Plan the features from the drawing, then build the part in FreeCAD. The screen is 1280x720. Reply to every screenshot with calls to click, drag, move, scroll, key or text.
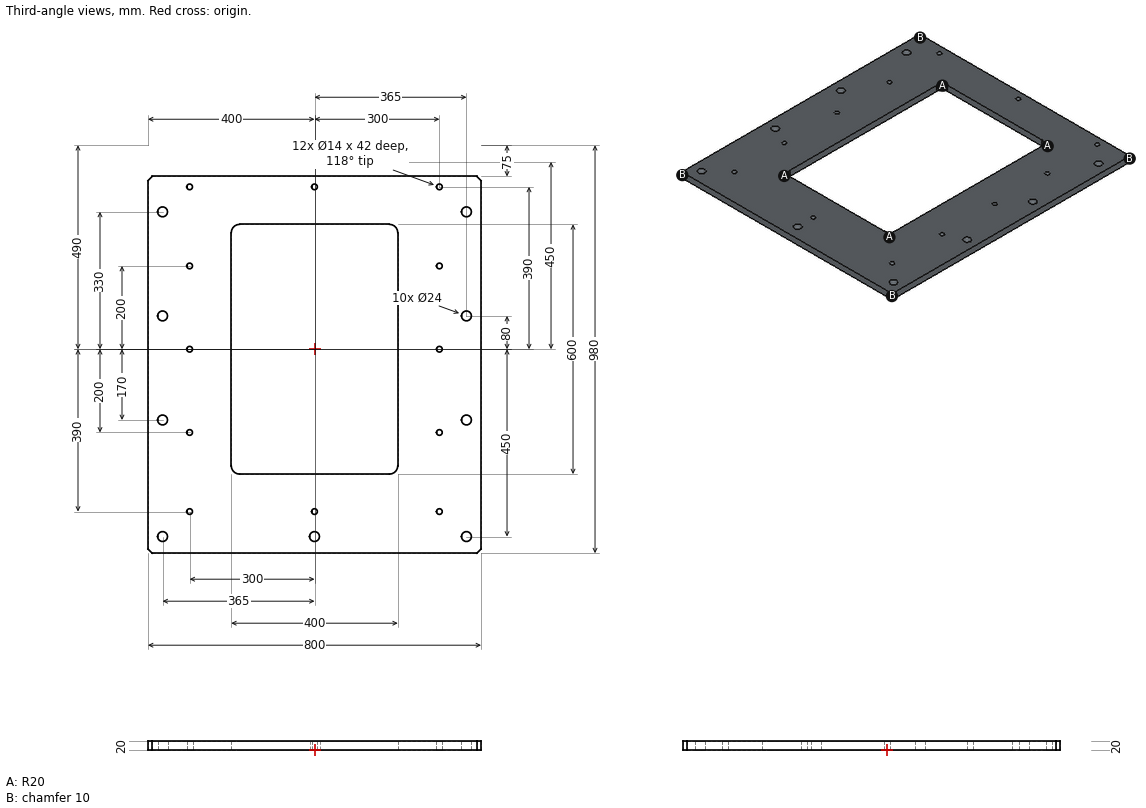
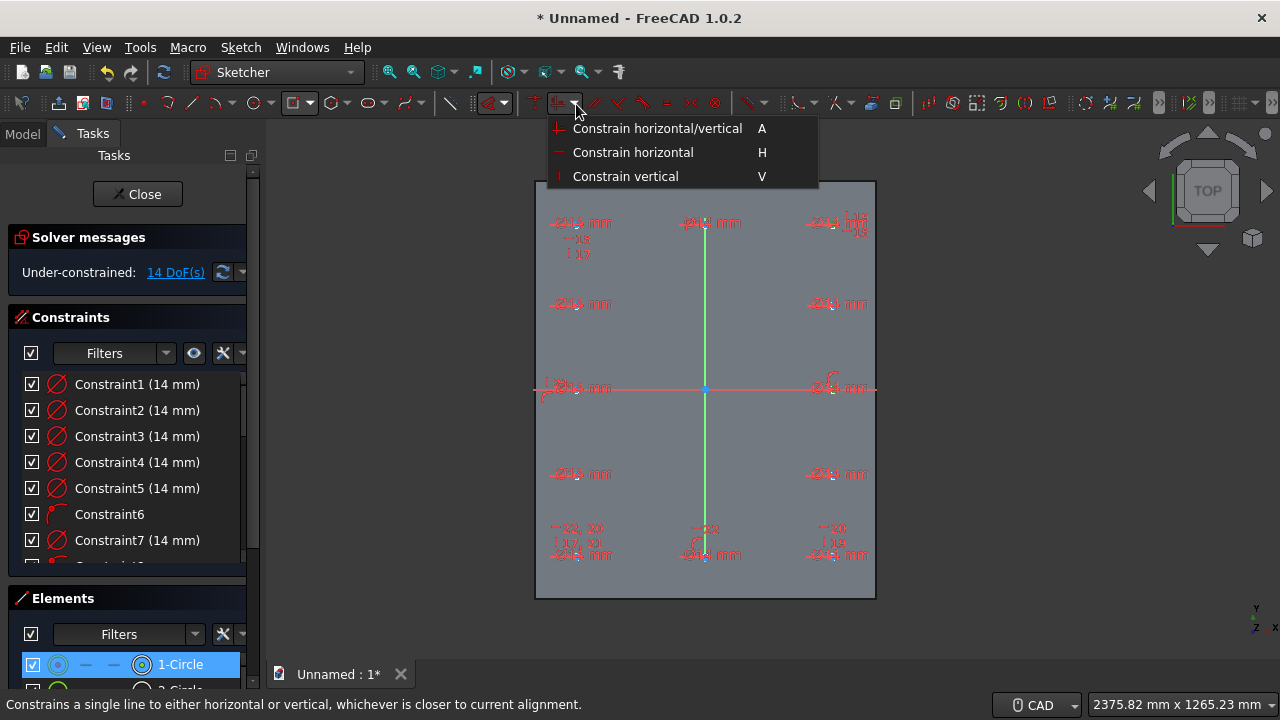
click(683, 176)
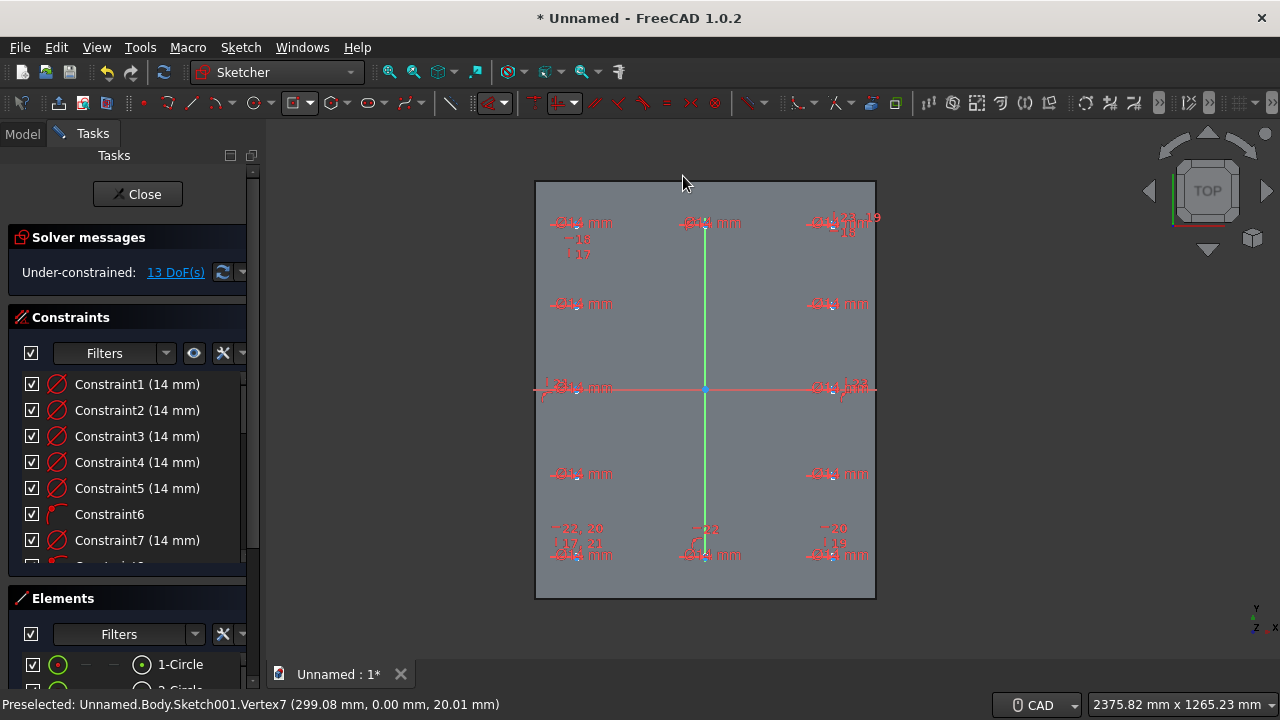
click(833, 225)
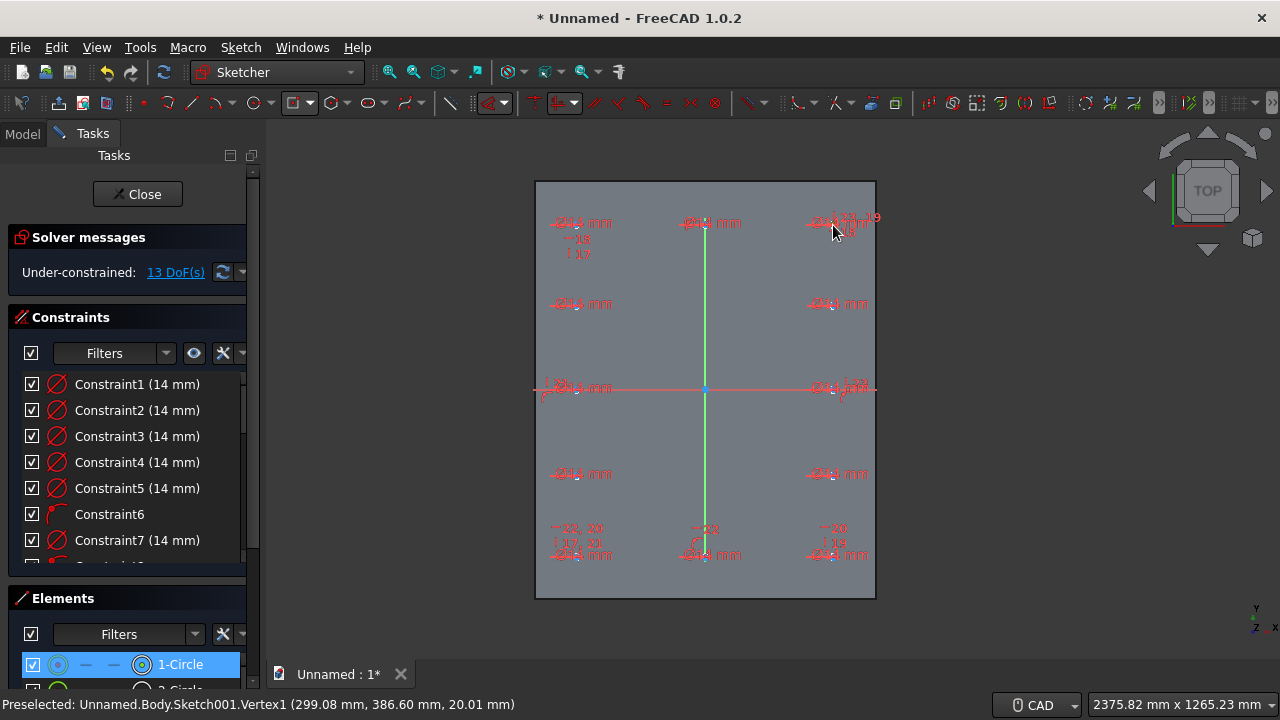
click(705, 225)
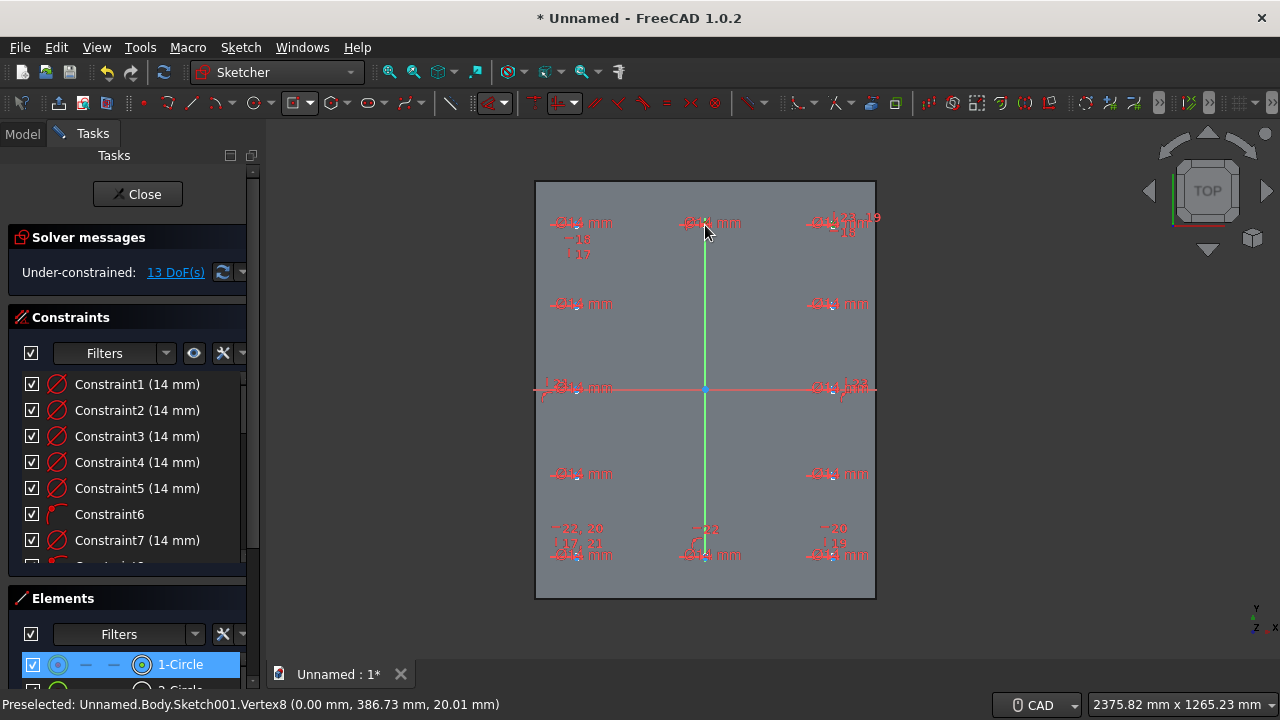
click(576, 104)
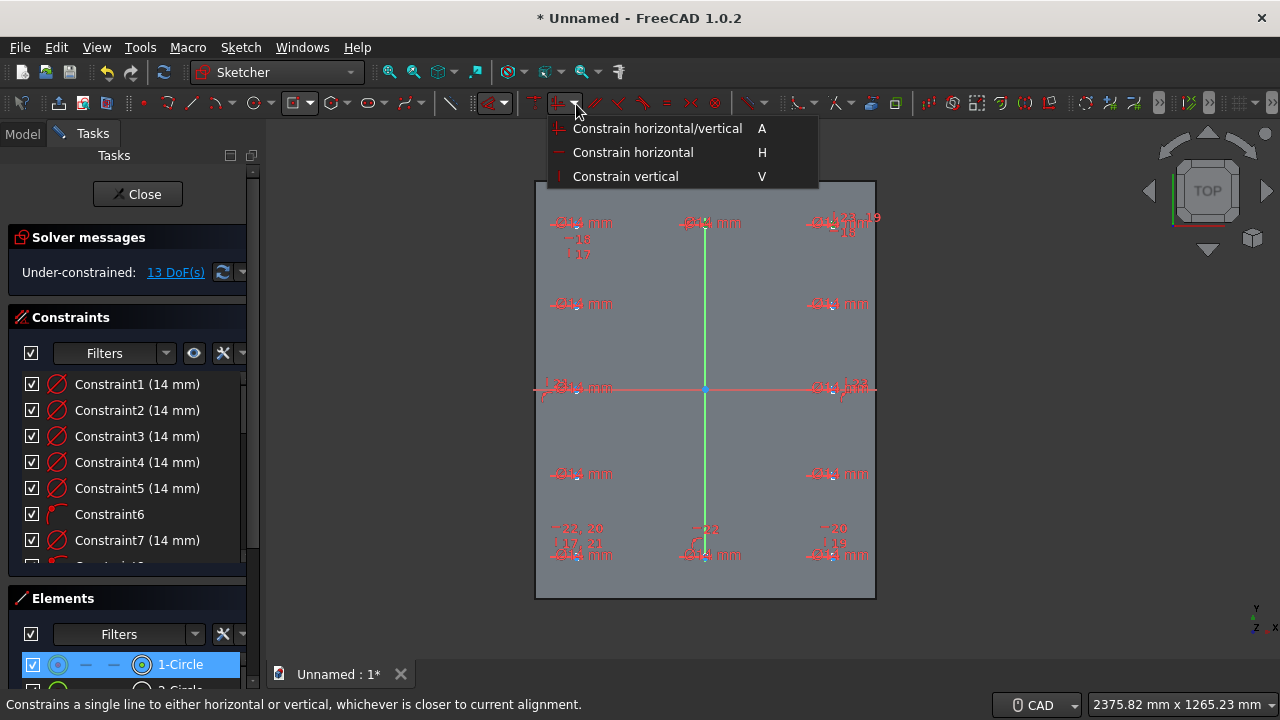
click(683, 152)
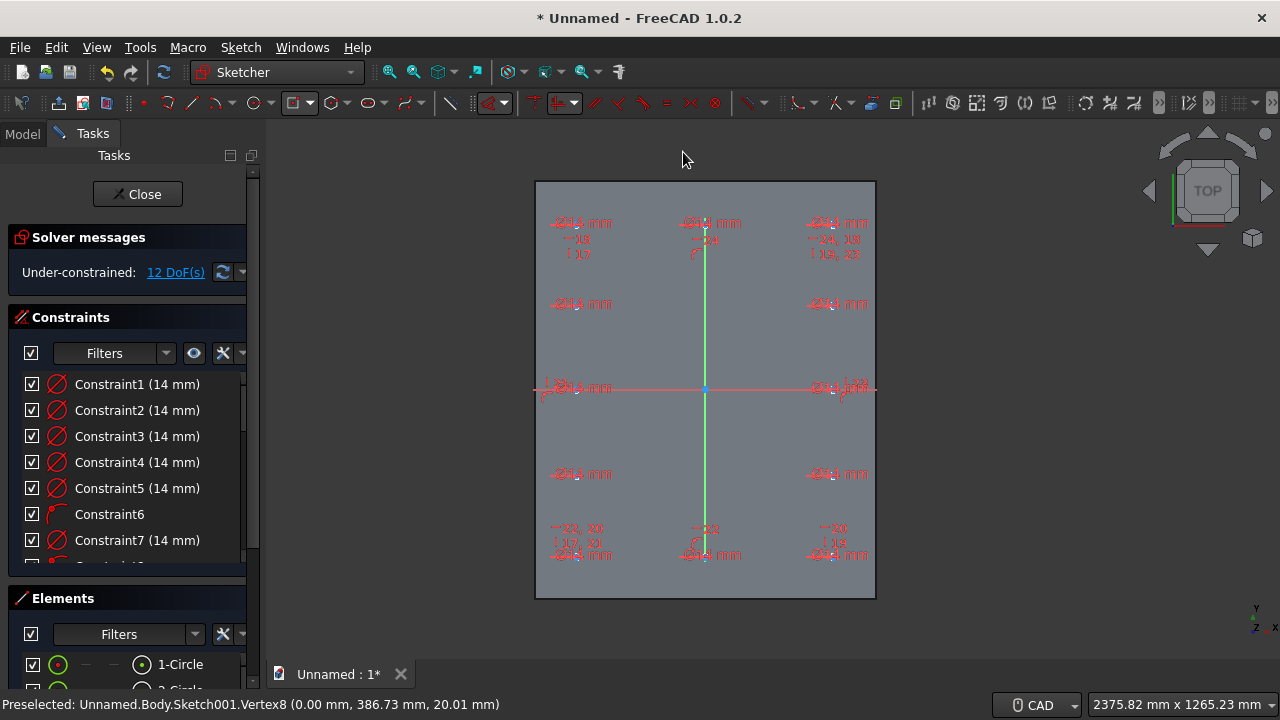
click(577, 225)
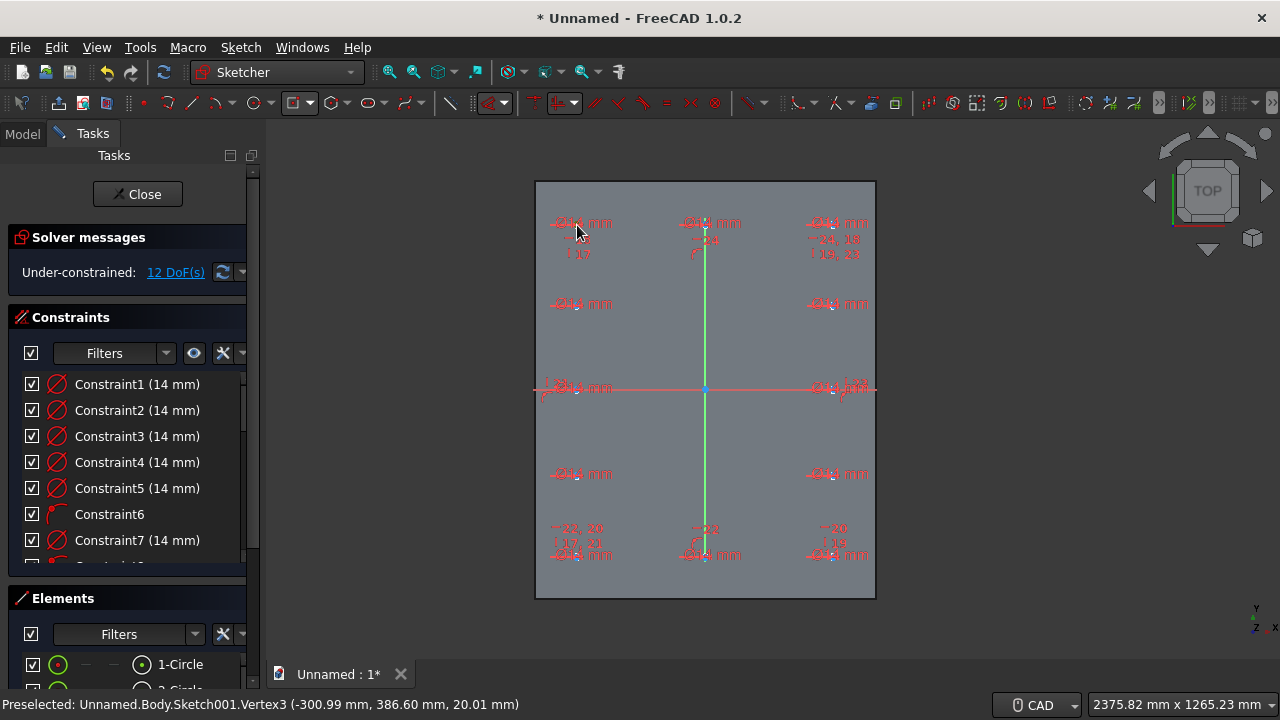
click(577, 306)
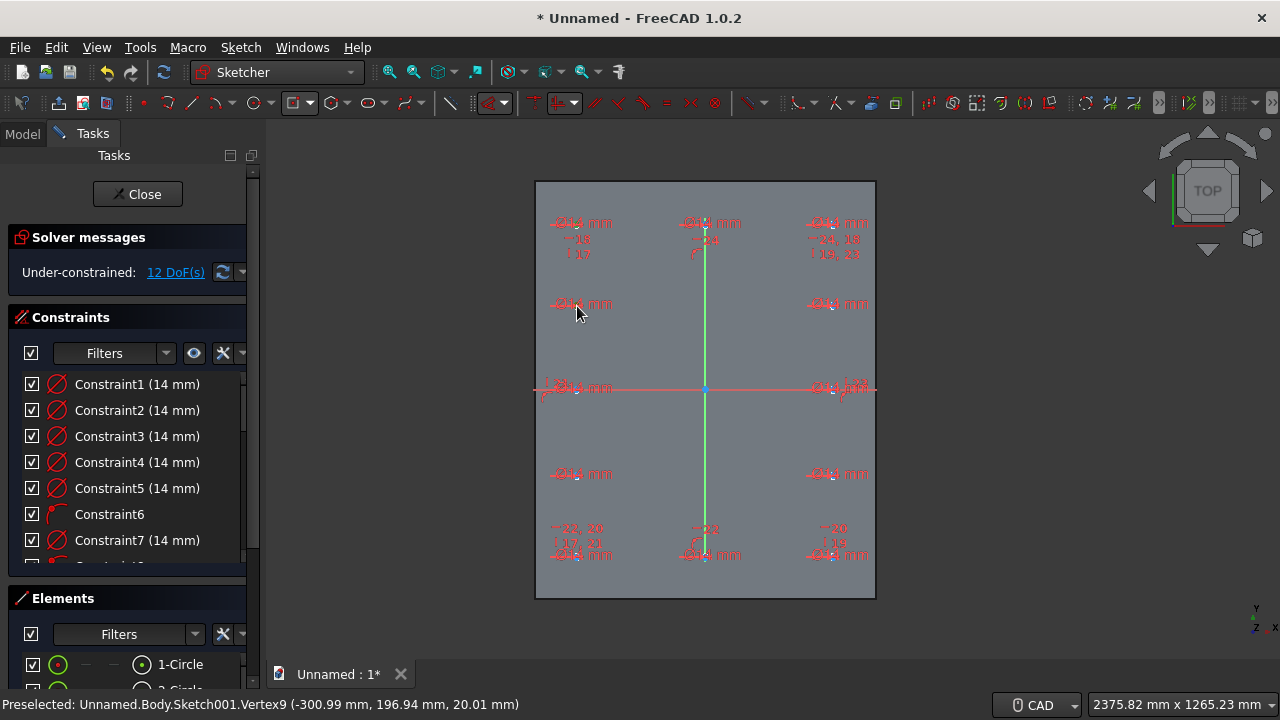
click(576, 104)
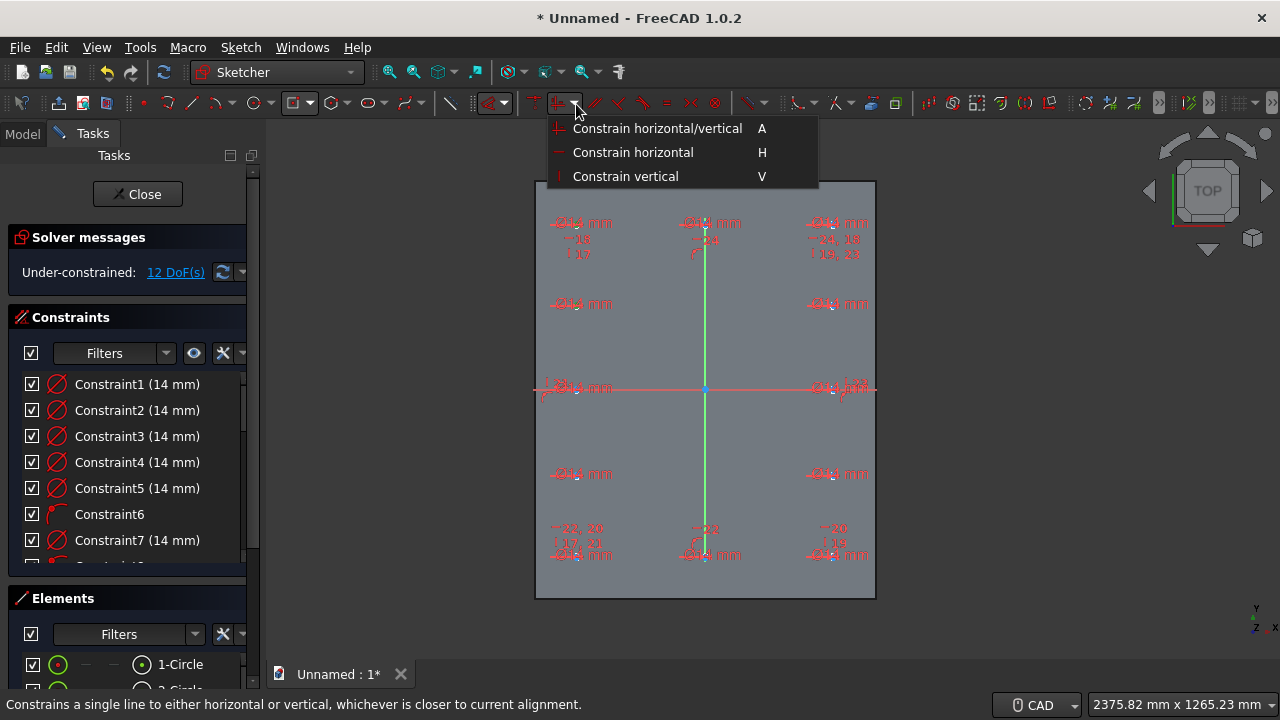
click(683, 176)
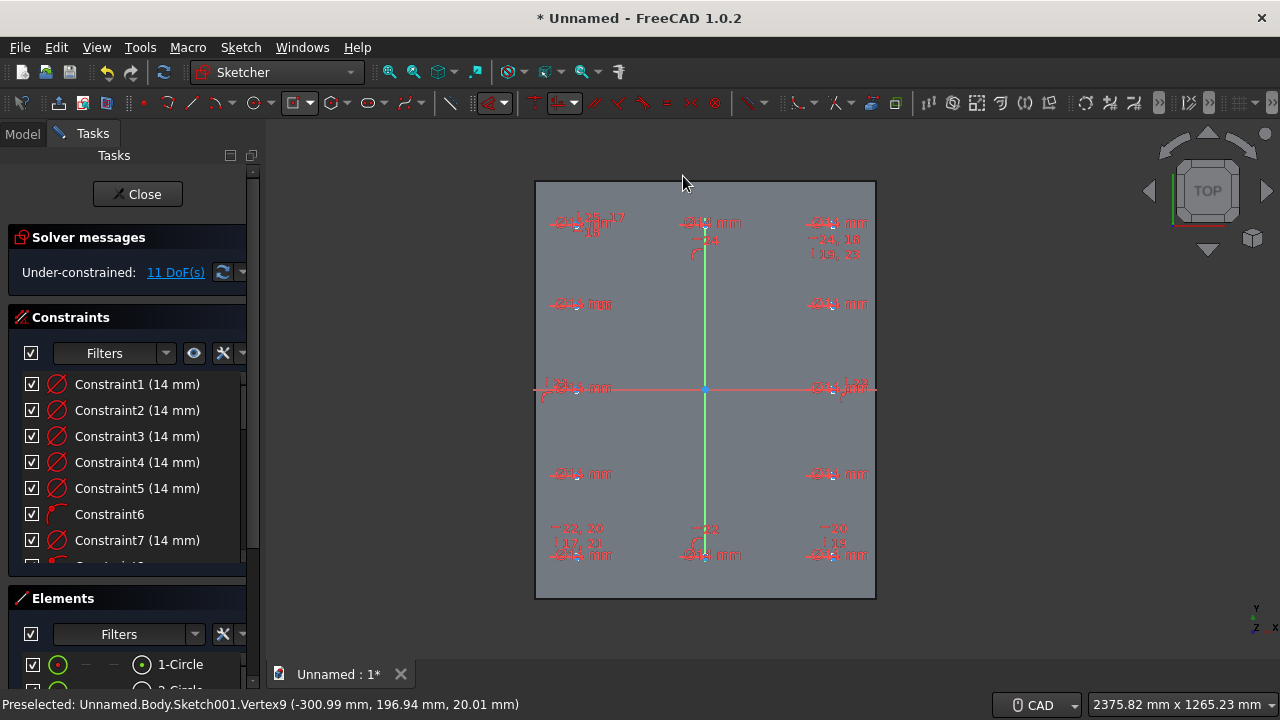
click(833, 225)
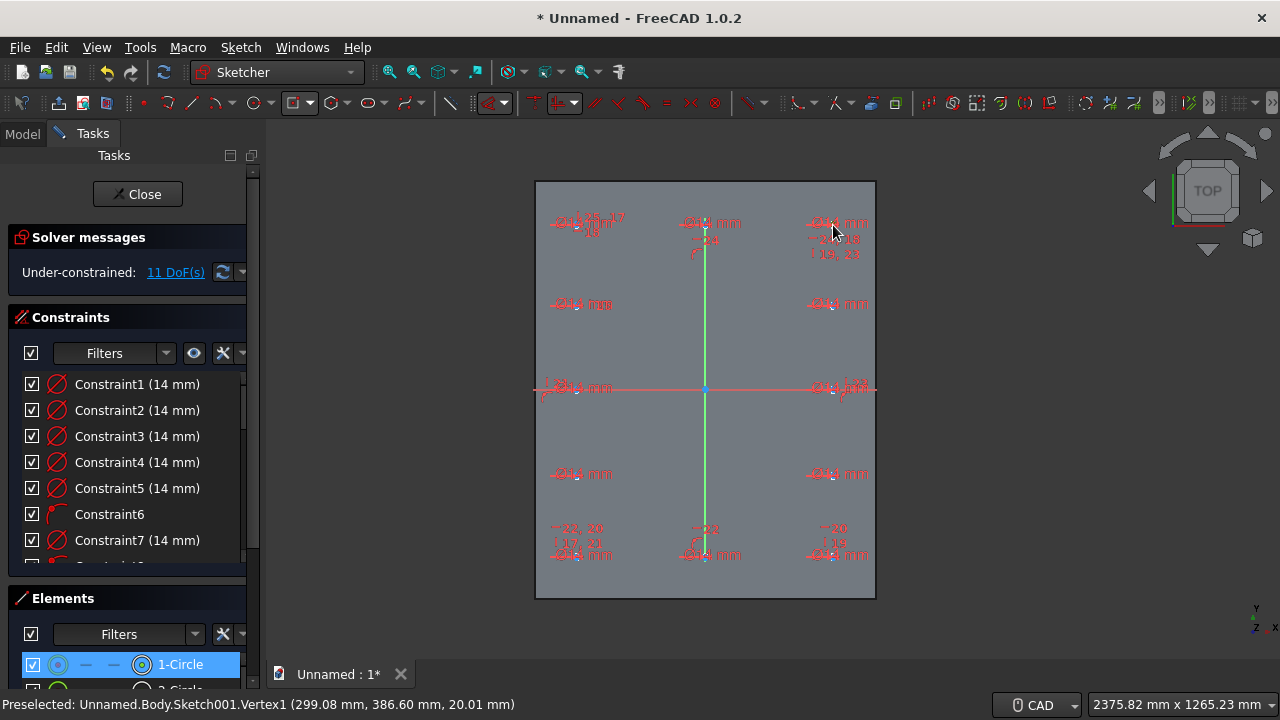
click(833, 306)